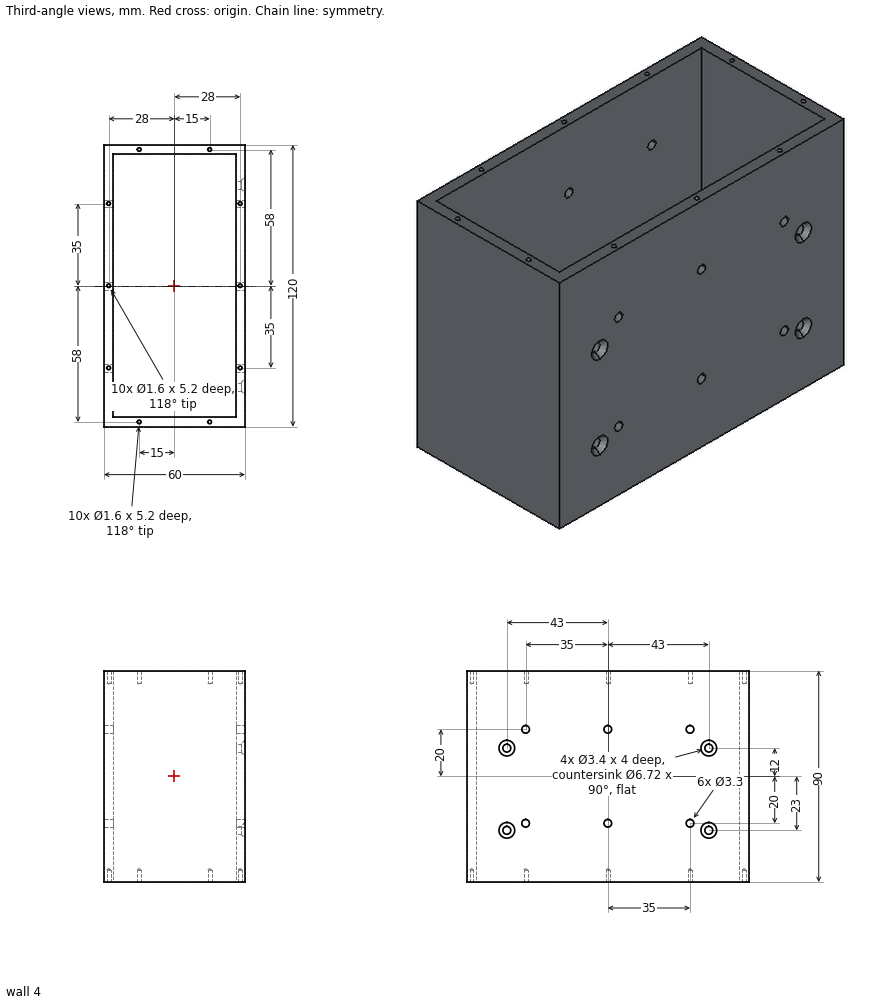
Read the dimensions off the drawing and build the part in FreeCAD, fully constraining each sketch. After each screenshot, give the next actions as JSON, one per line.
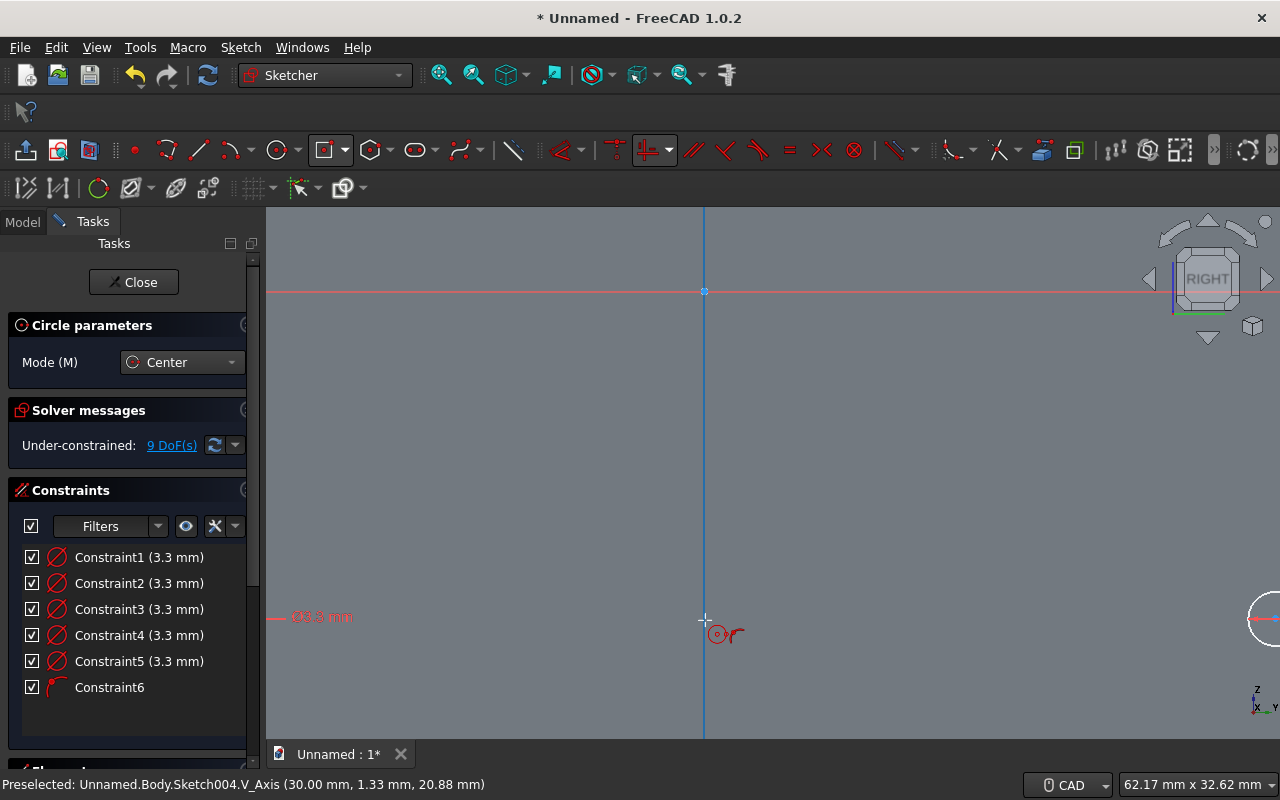
{"action": "left_click", "coordinate": [704, 618]}
{"action": "mouse_move", "coordinate": [723, 599]}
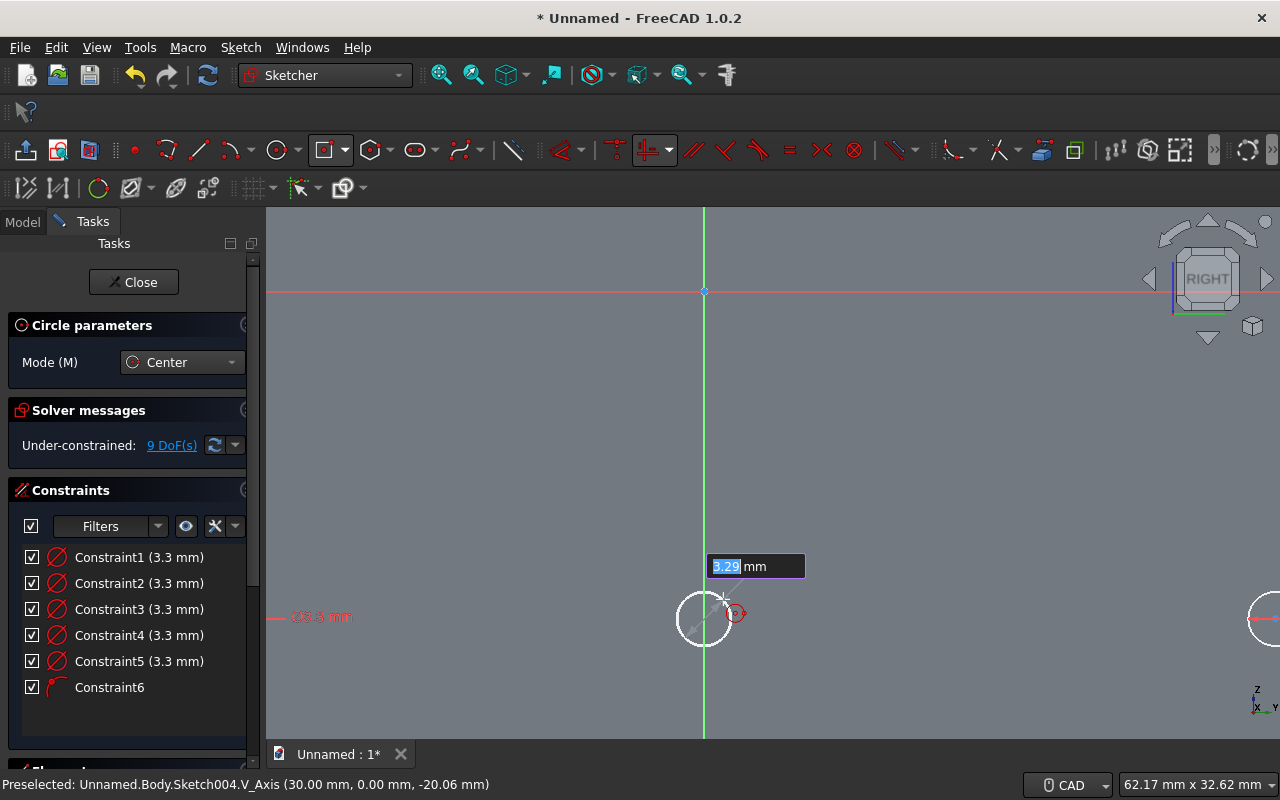
{"action": "type", "text": "3.3"}
{"action": "key", "text": "Return"}
{"action": "key", "text": "Escape"}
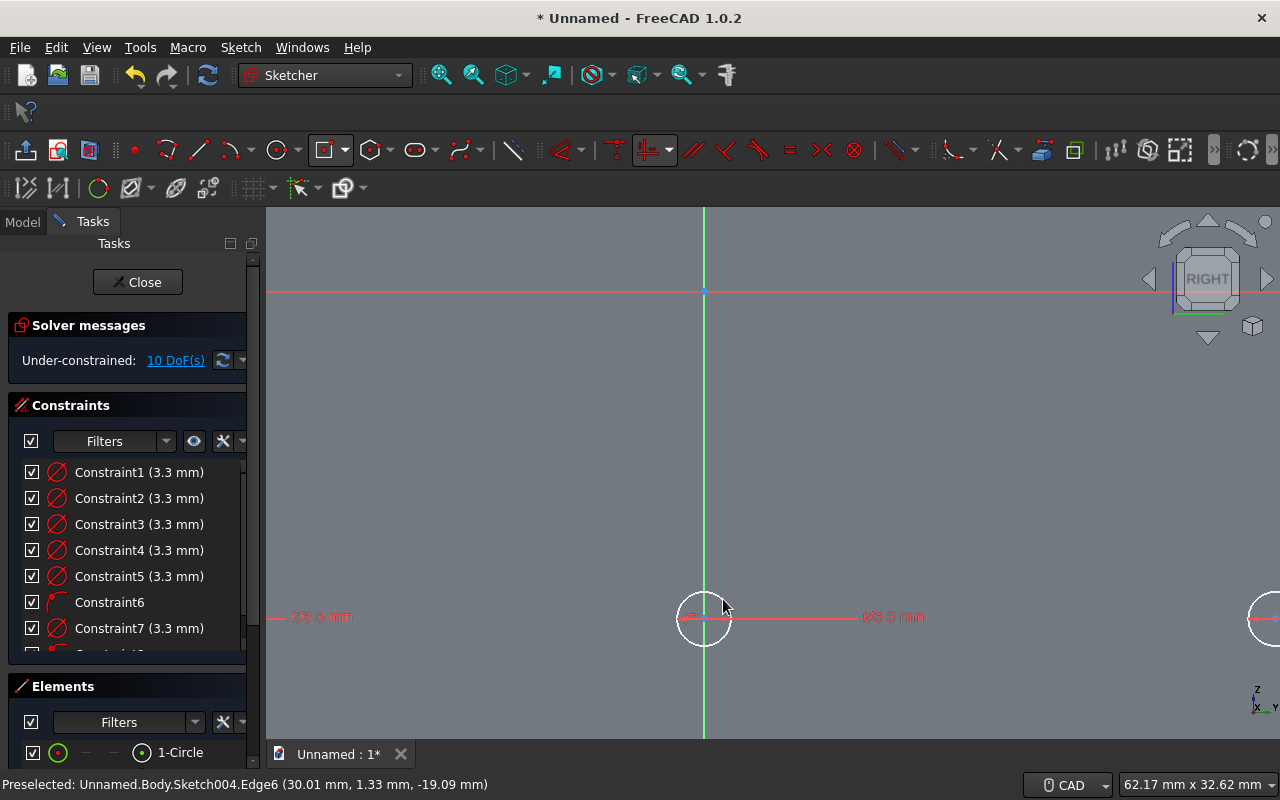
{"action": "scroll", "coordinate": [705, 621], "scroll_direction": "down", "scroll_amount": 4}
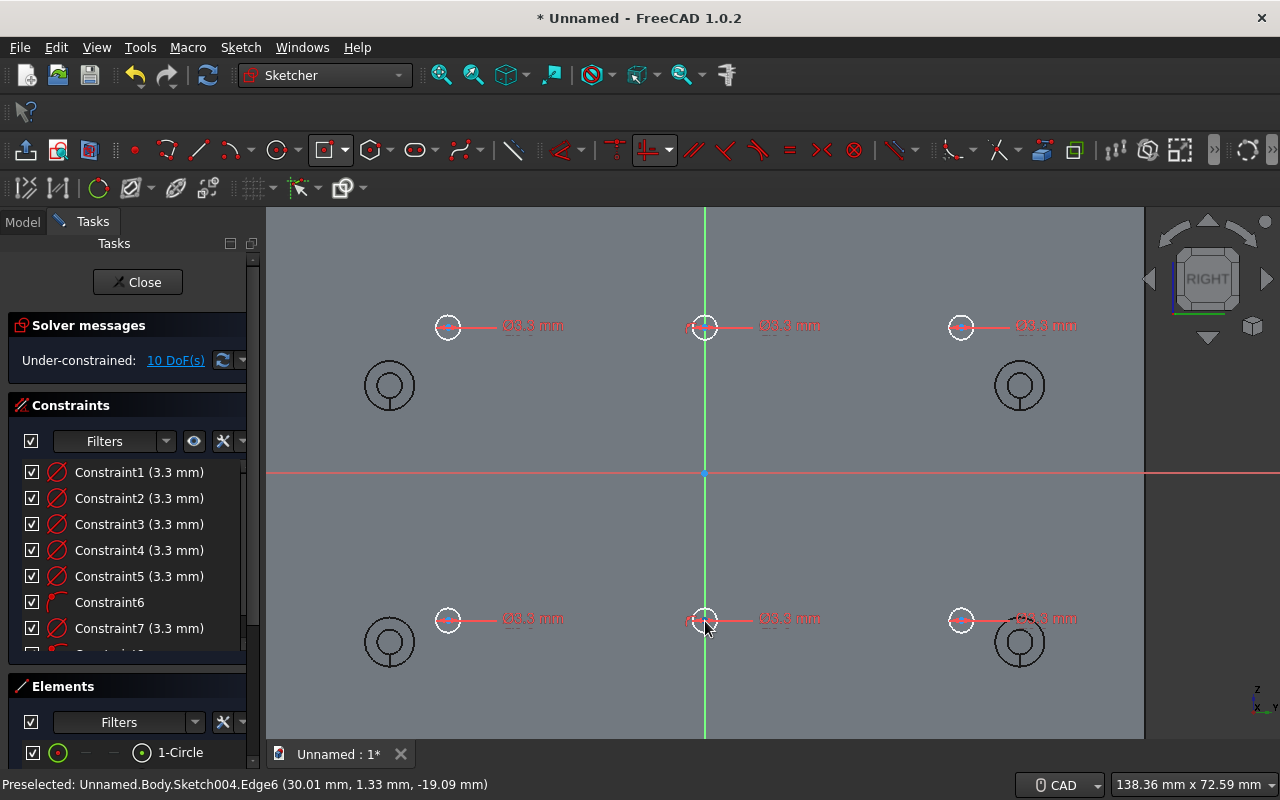
{"action": "left_click", "coordinate": [961, 621]}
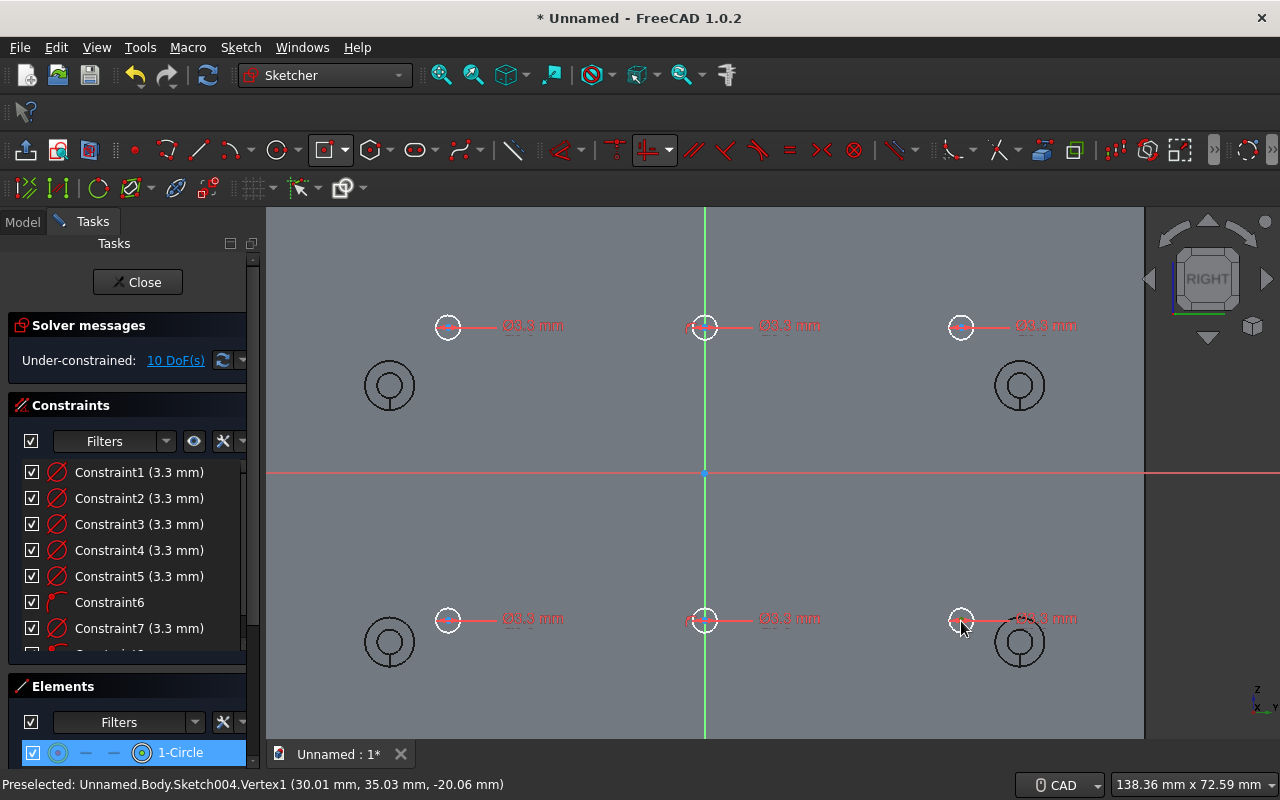
{"action": "left_click", "coordinate": [961, 328]}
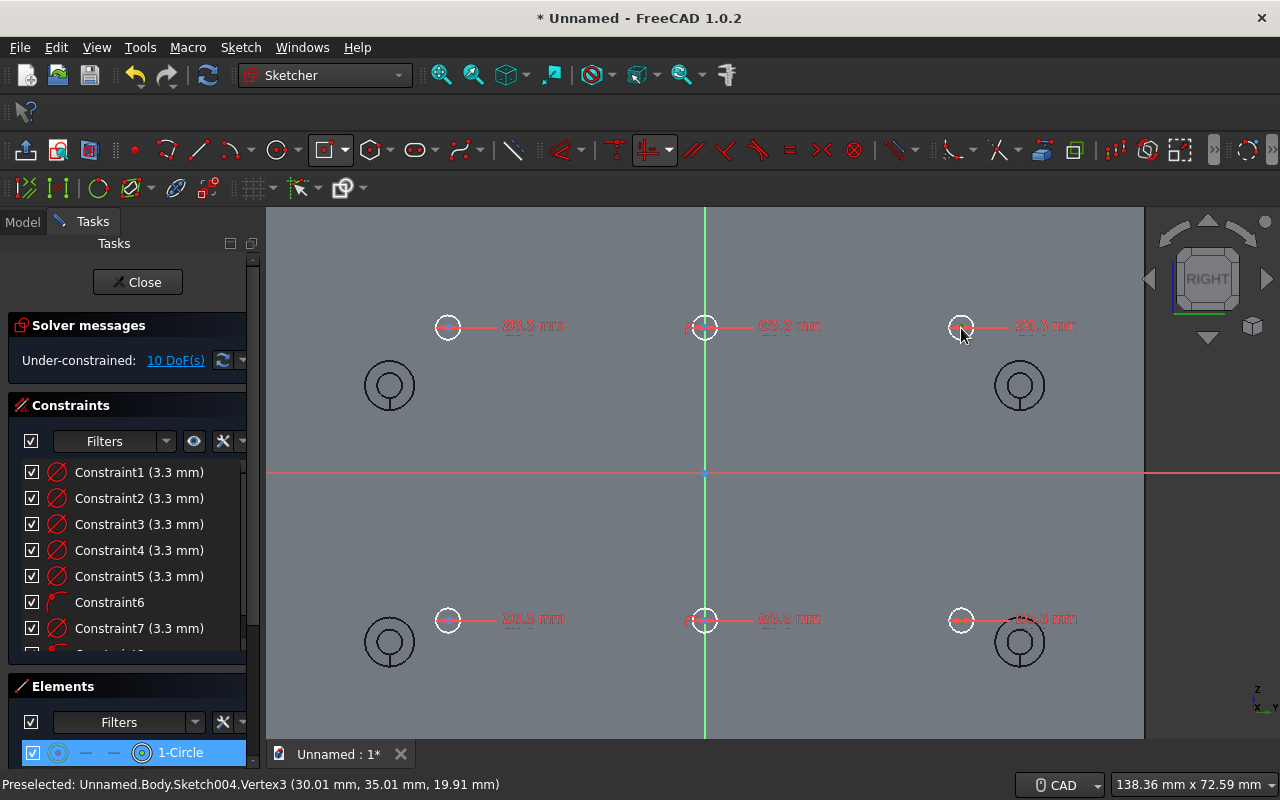
{"action": "left_click", "coordinate": [672, 150]}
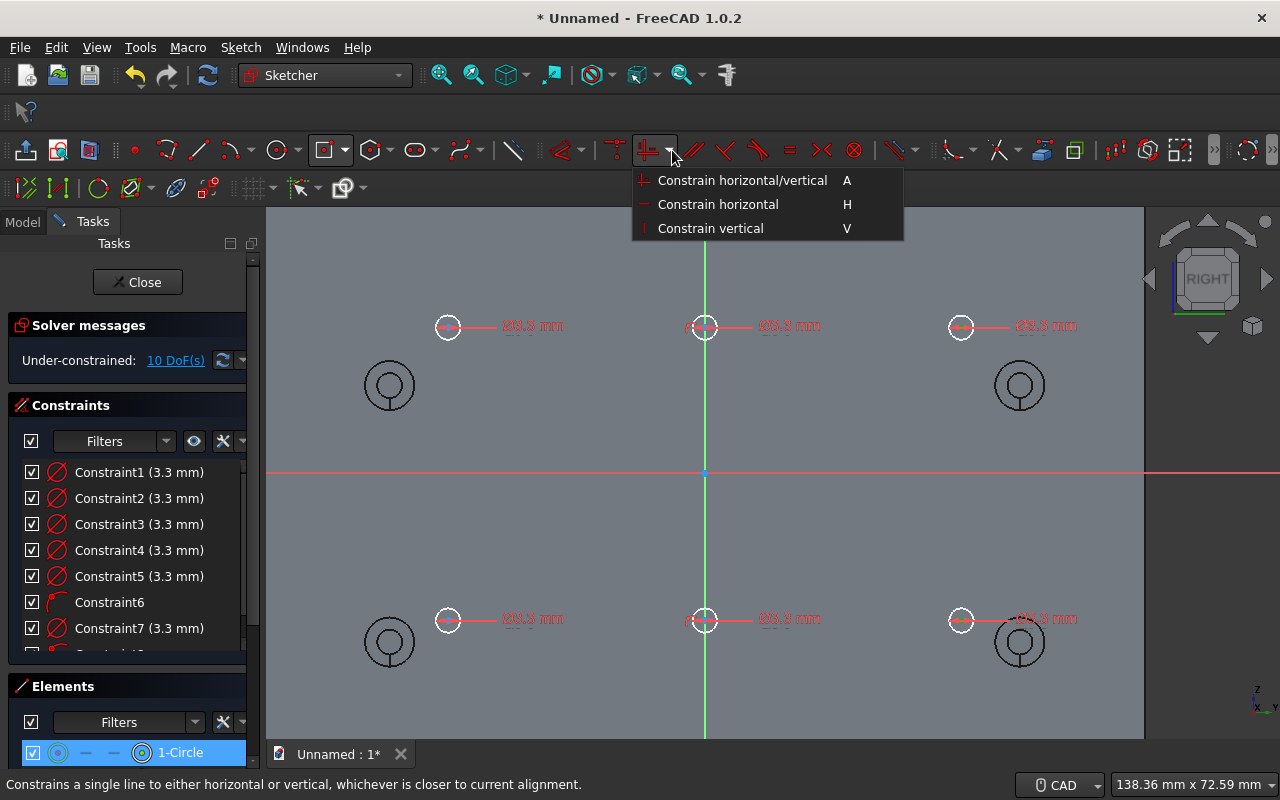
{"action": "left_click", "coordinate": [768, 228]}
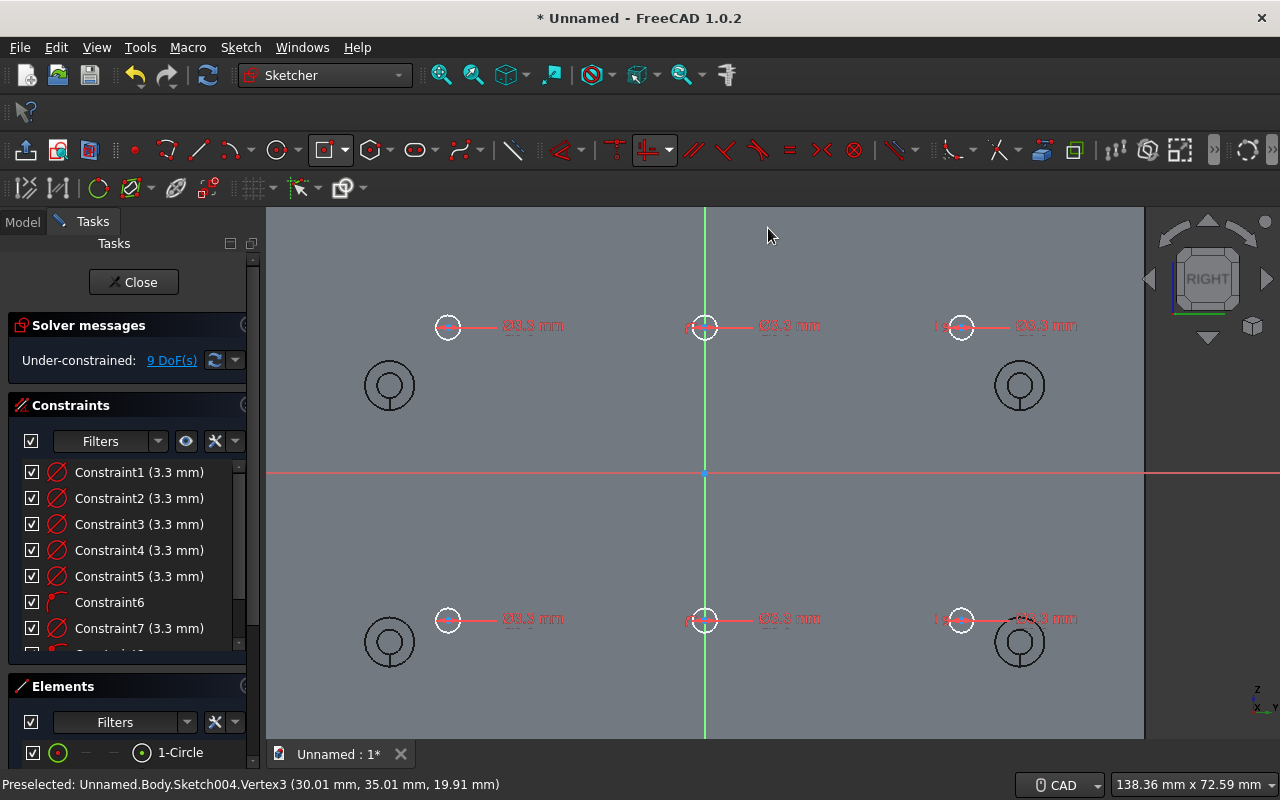
{"action": "left_click", "coordinate": [448, 328]}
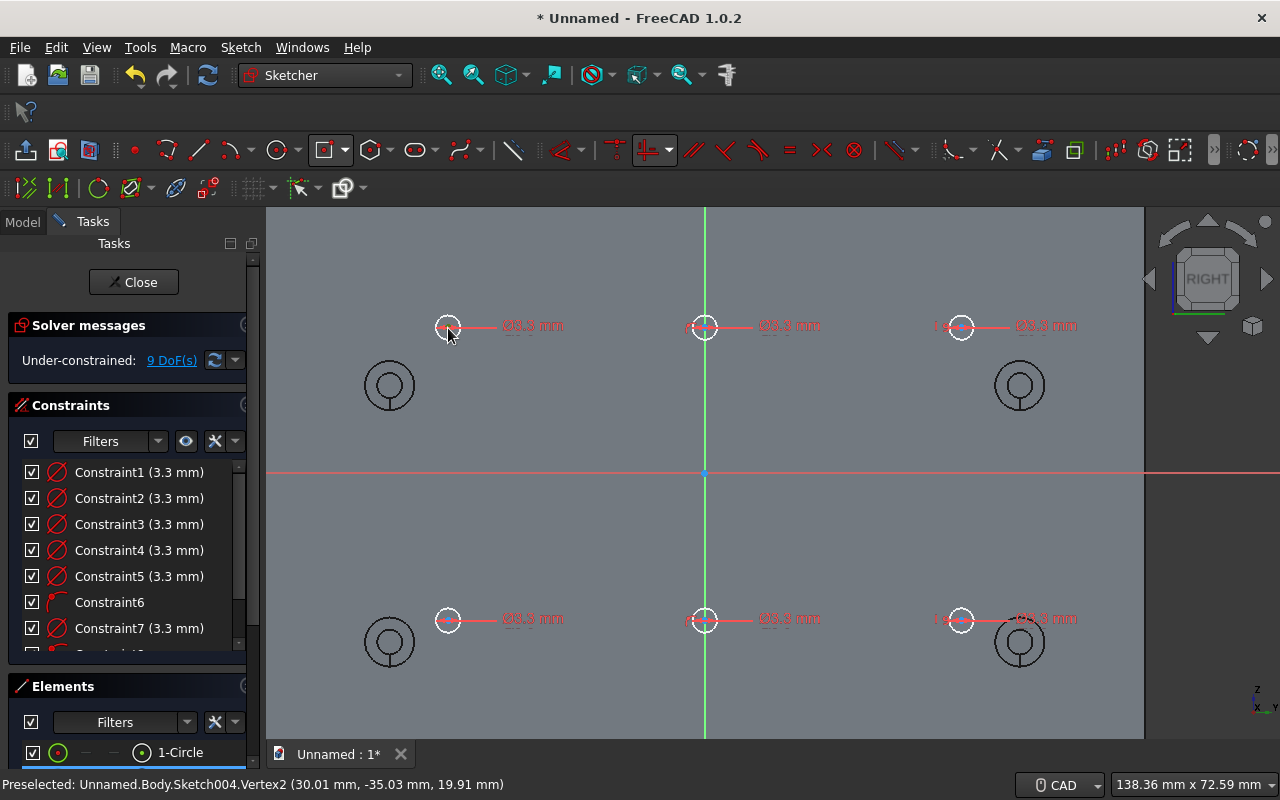
{"action": "left_click", "coordinate": [961, 328]}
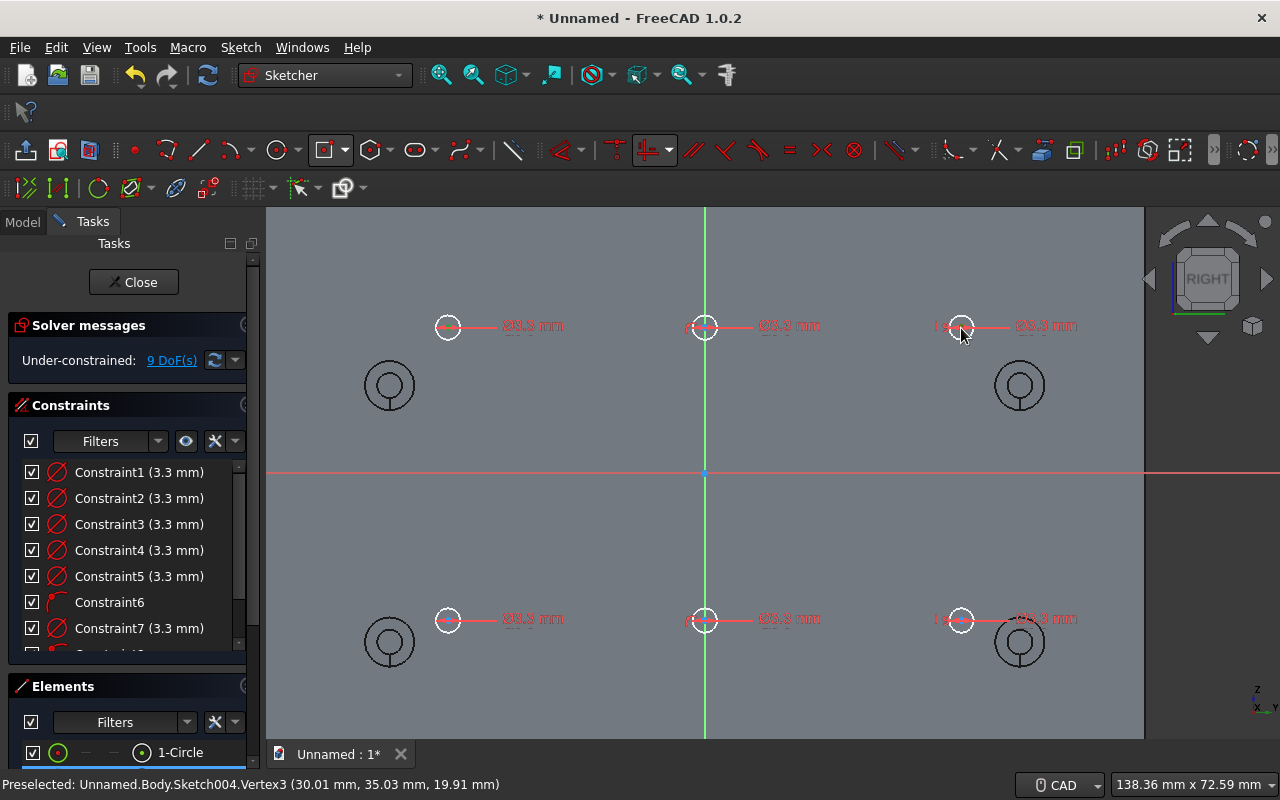
{"action": "key", "text": "h"}